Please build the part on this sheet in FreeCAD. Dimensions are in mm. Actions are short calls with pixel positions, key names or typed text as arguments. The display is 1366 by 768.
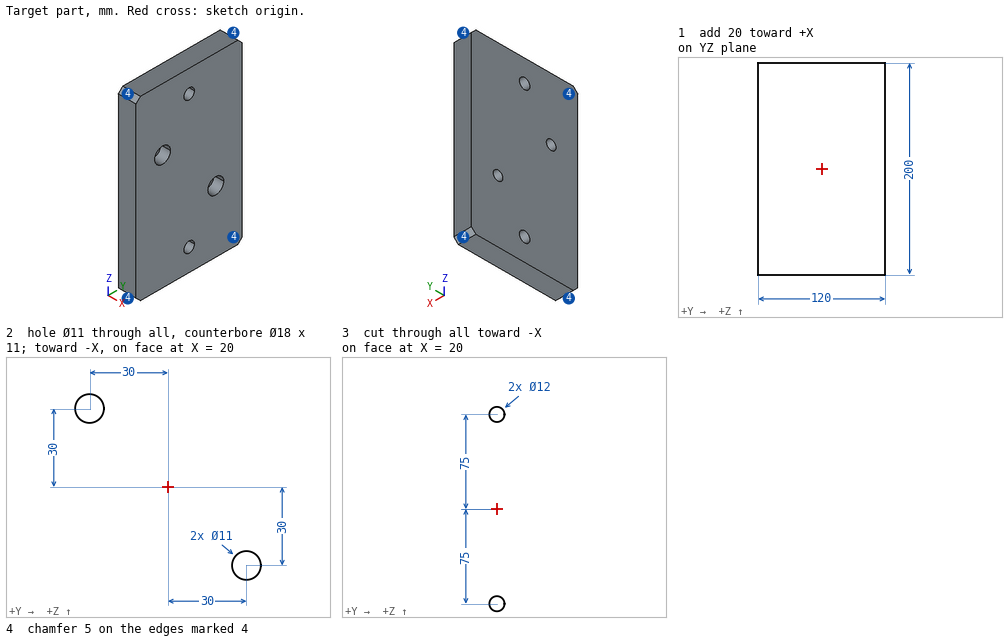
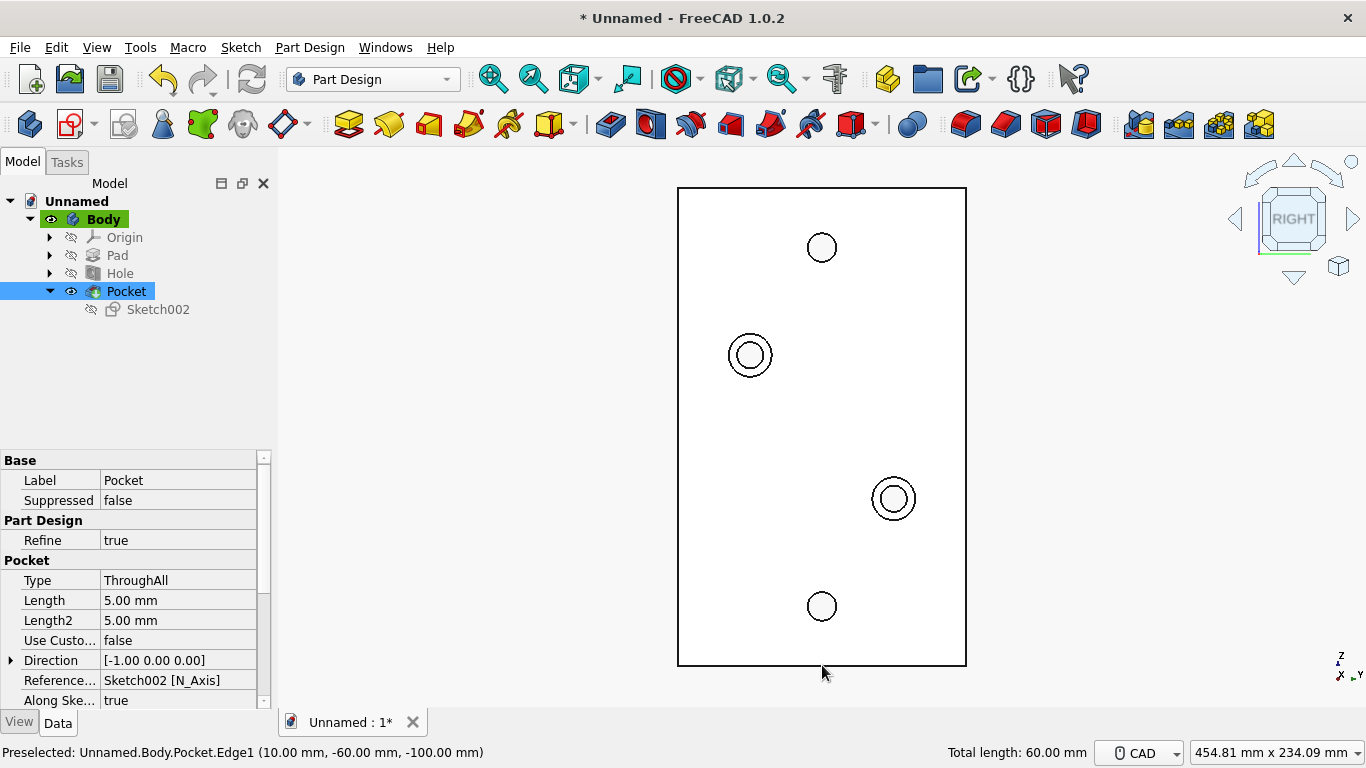
key(5)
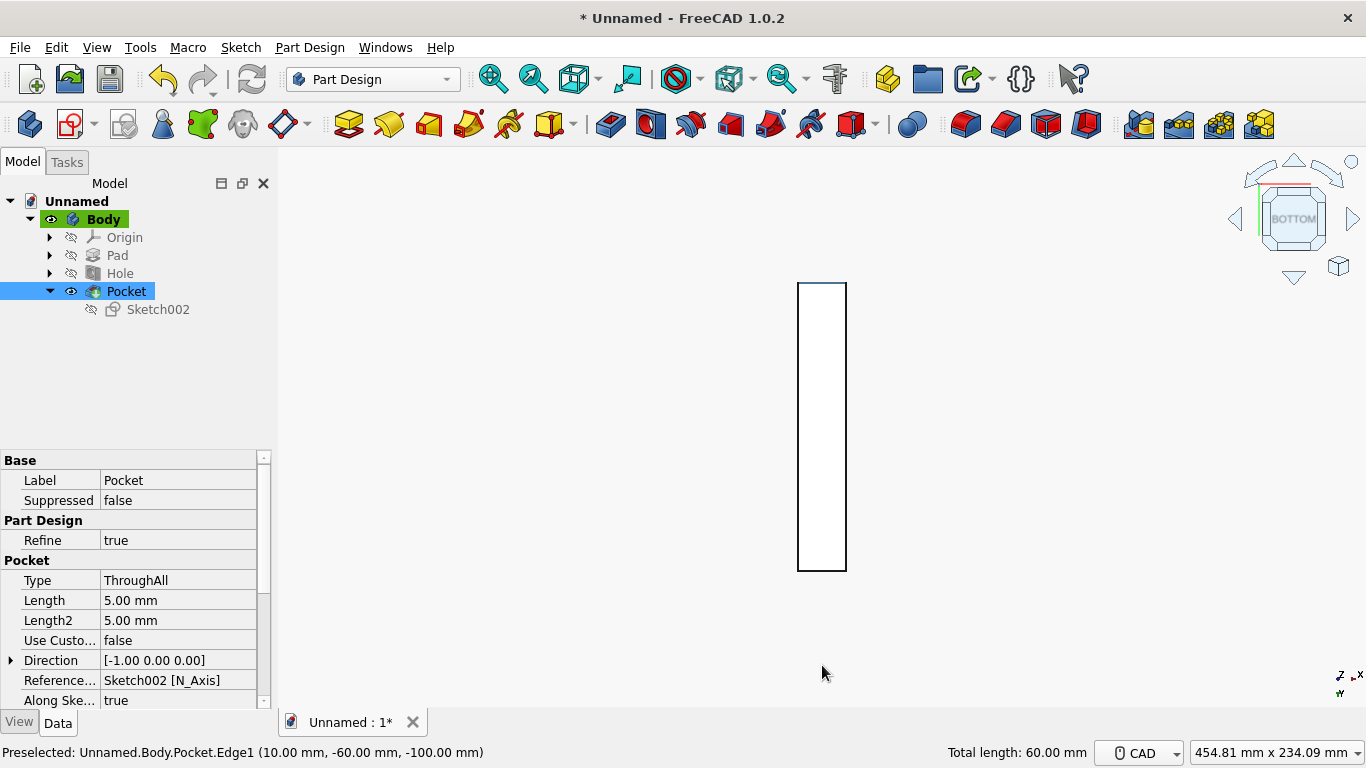
click(822, 570, ctrl)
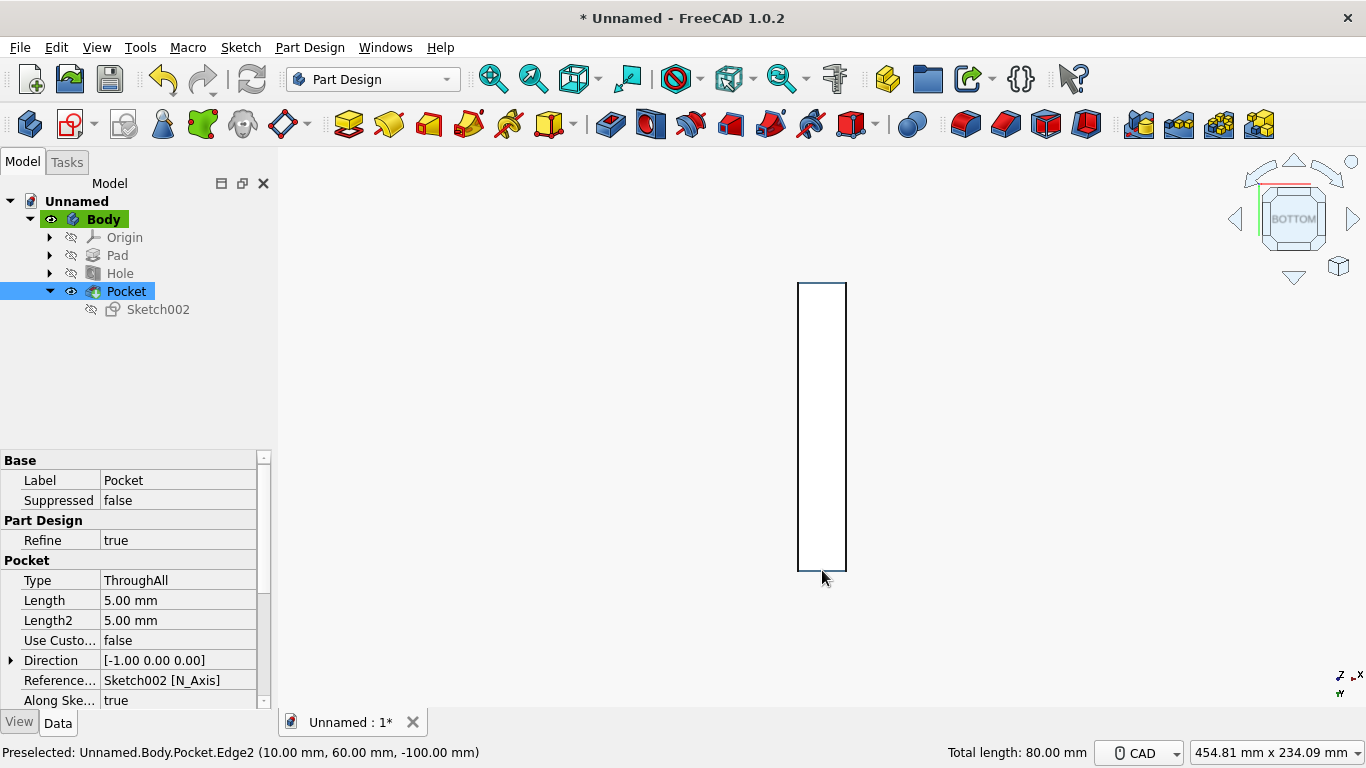
click(1006, 124)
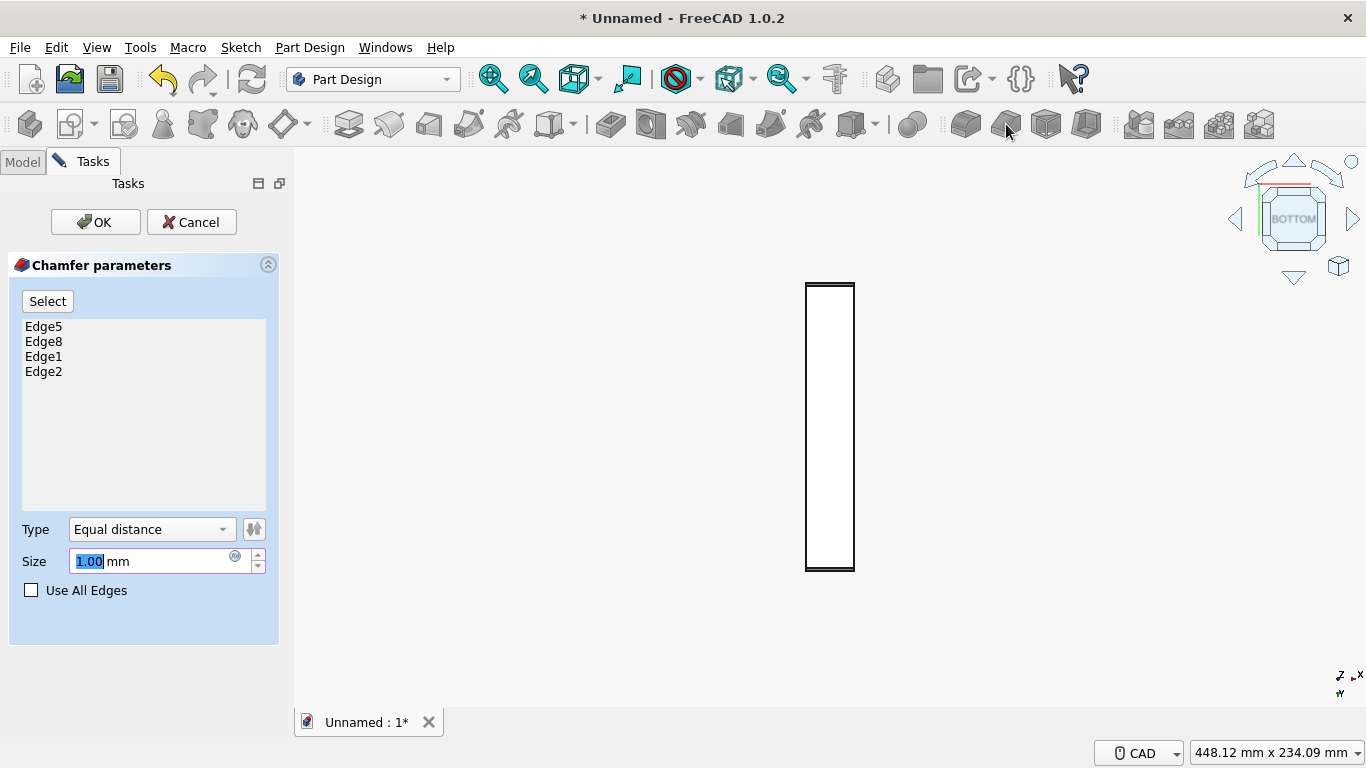
text(5)
key(Tab)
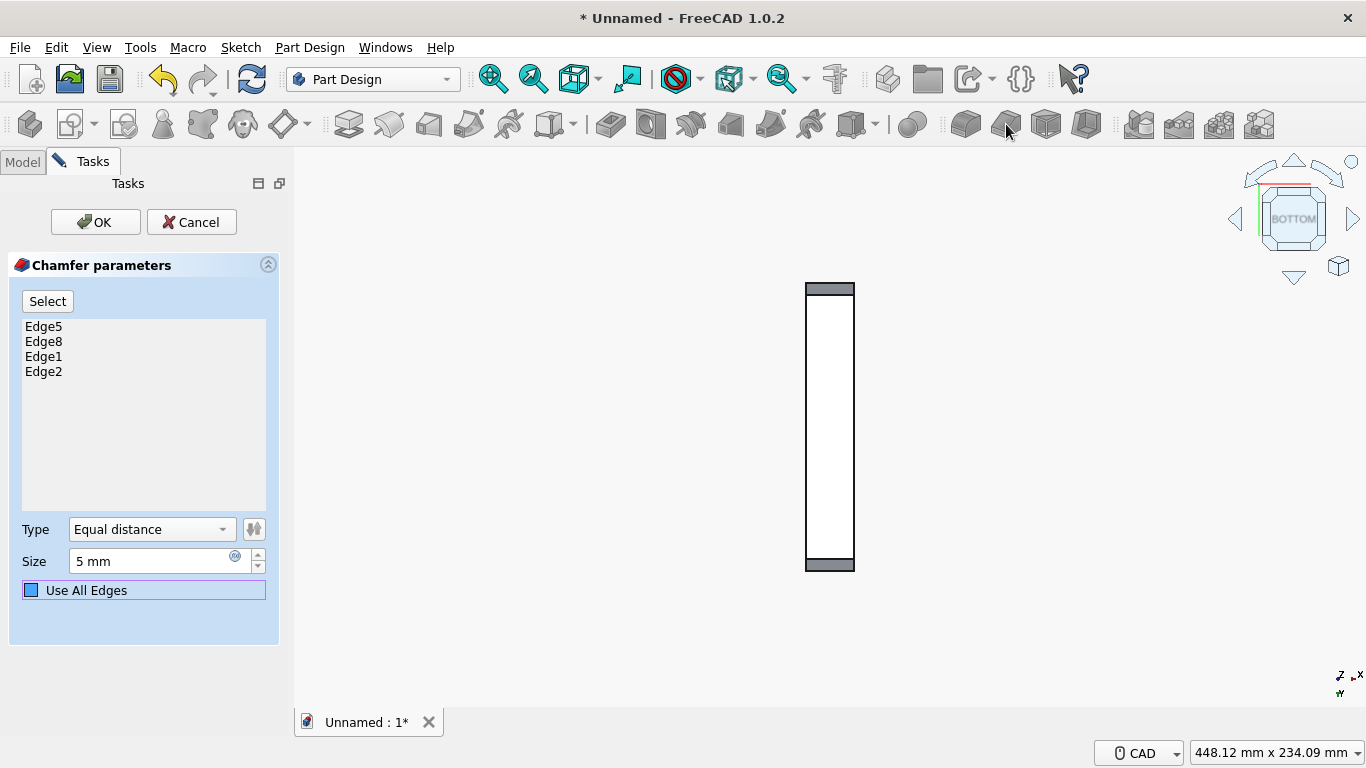
click(96, 222)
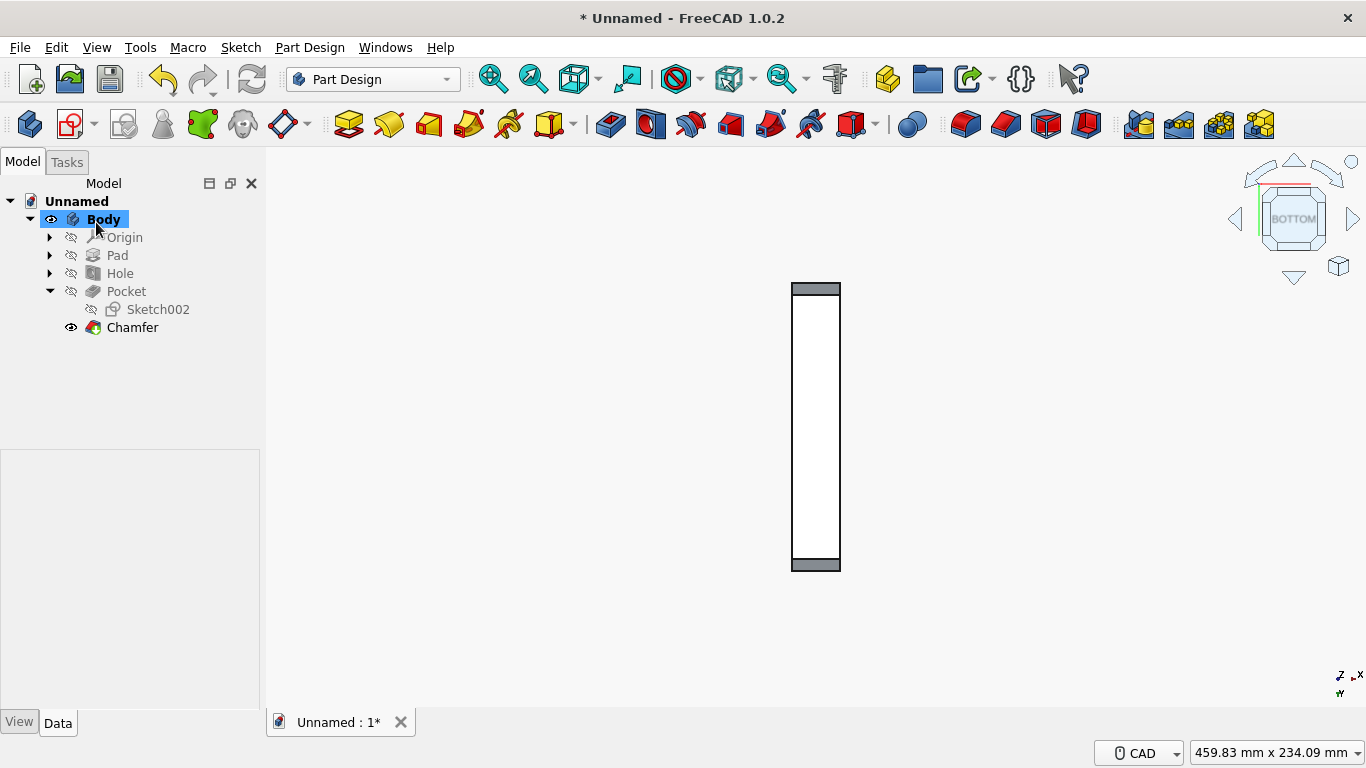
key(0)